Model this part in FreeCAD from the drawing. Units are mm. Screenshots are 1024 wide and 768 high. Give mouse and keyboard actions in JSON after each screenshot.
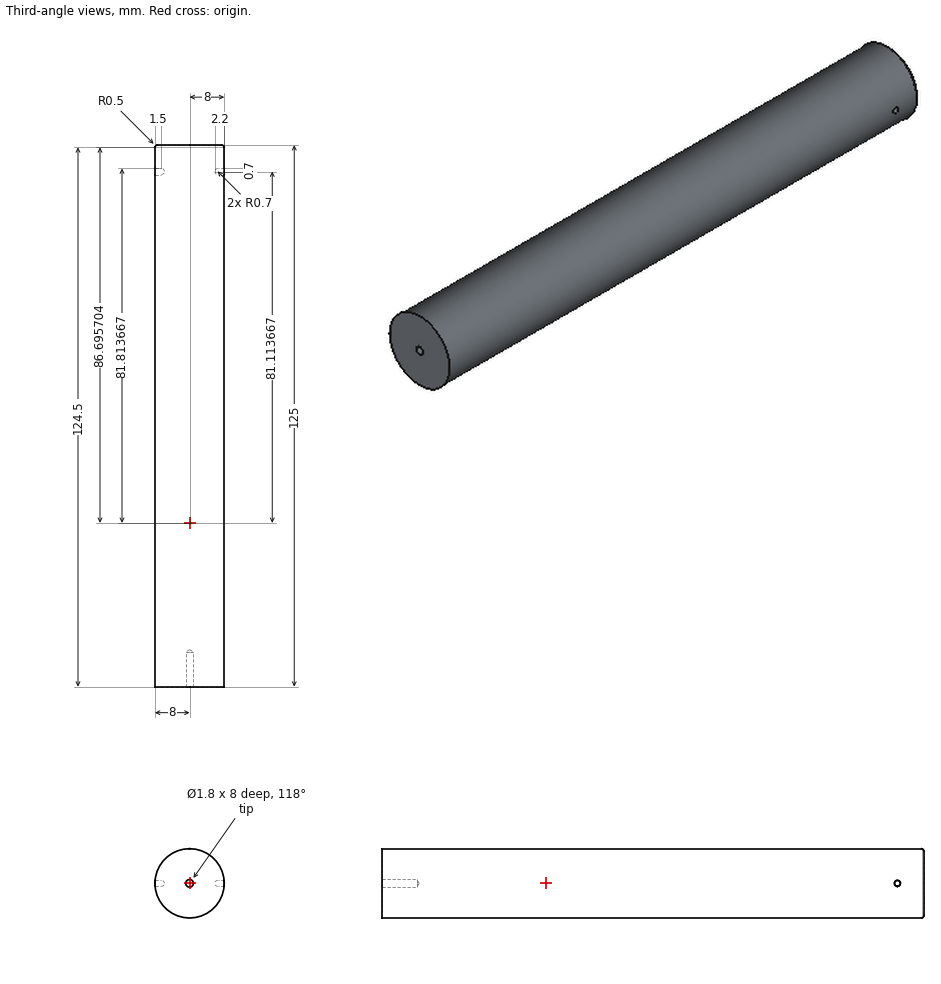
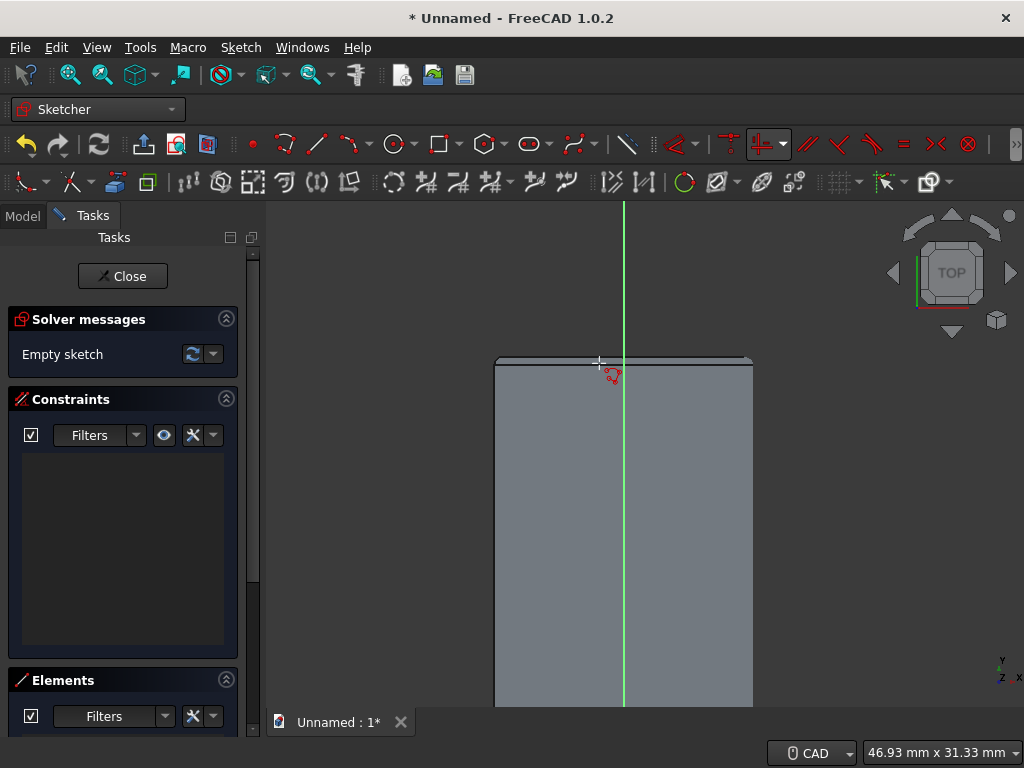
{"action": "left_click", "coordinate": [717, 455]}
{"action": "left_click", "coordinate": [753, 455]}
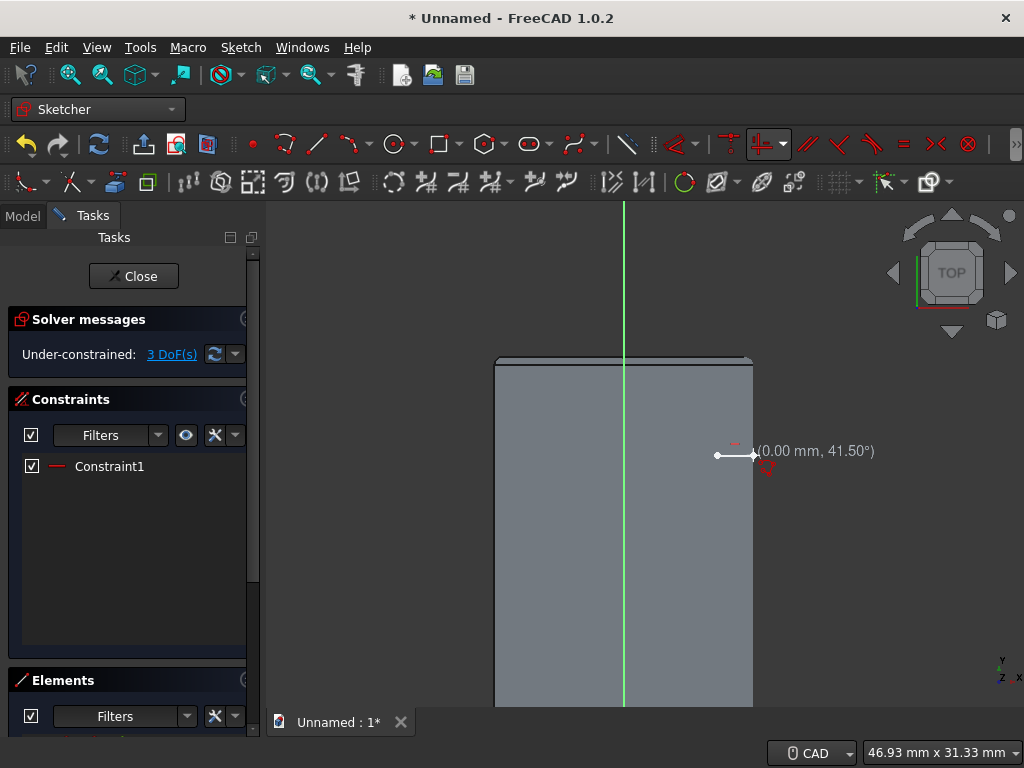
{"action": "scroll", "coordinate": [753, 444], "scroll_direction": "up", "scroll_amount": 2}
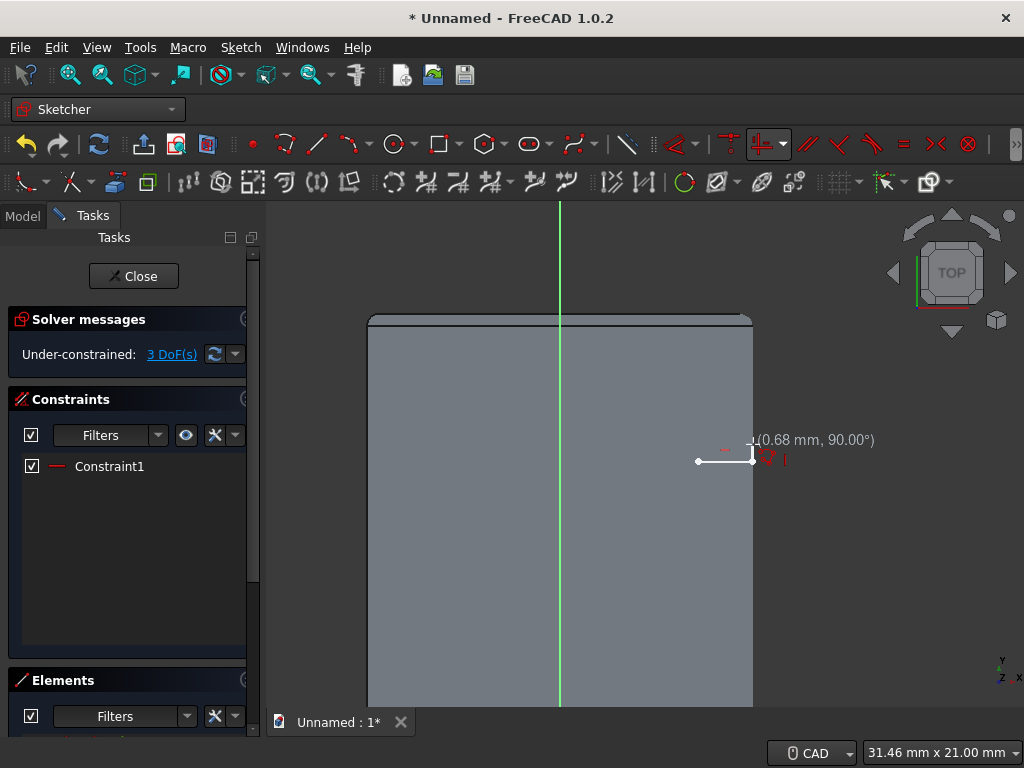
{"action": "left_click", "coordinate": [753, 443]}
{"action": "left_click", "coordinate": [716, 443]}
{"action": "right_click", "coordinate": [716, 443]}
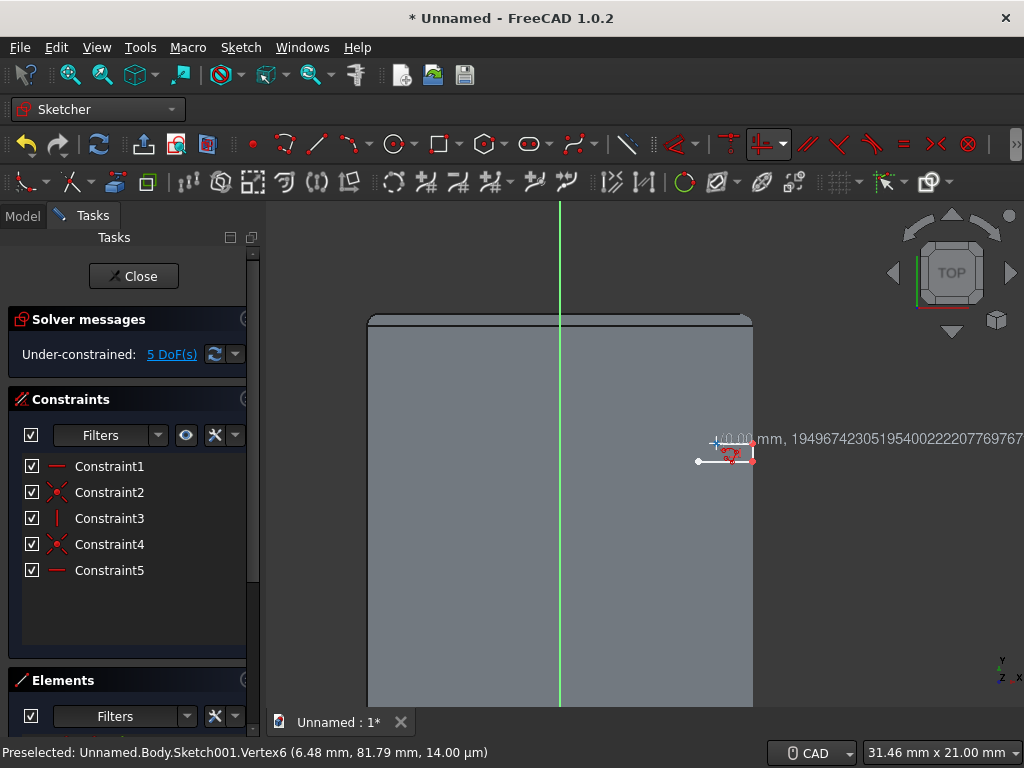
{"action": "key", "text": "g 3 a"}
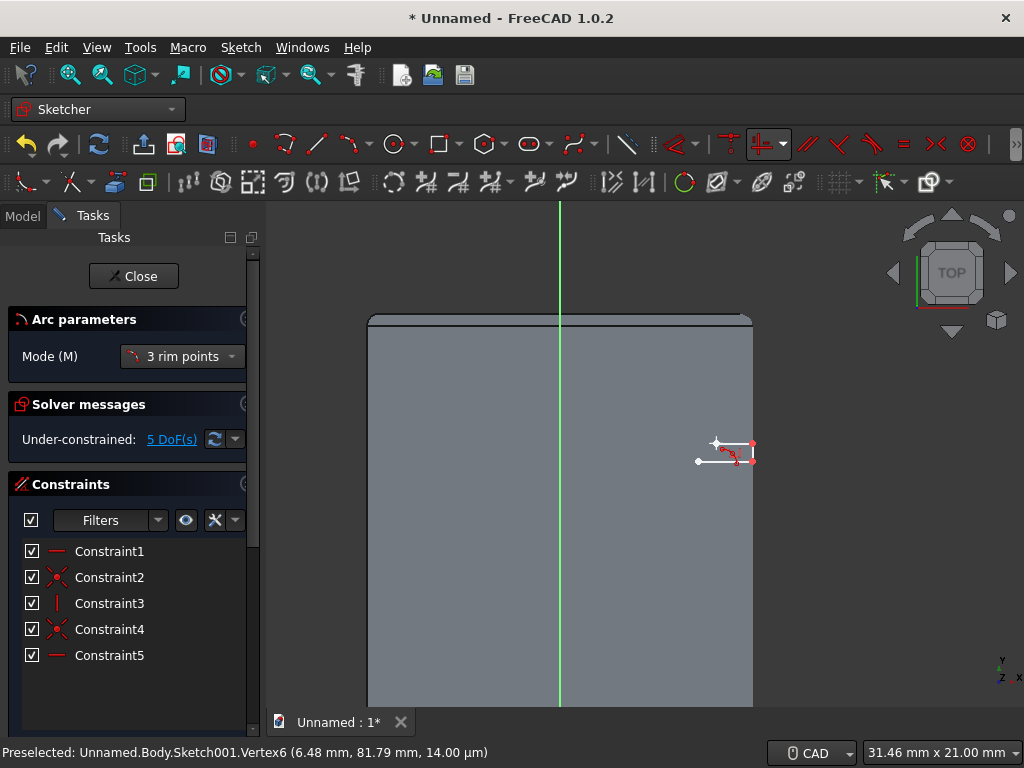
{"action": "left_click", "coordinate": [716, 444]}
{"action": "left_click", "coordinate": [699, 462]}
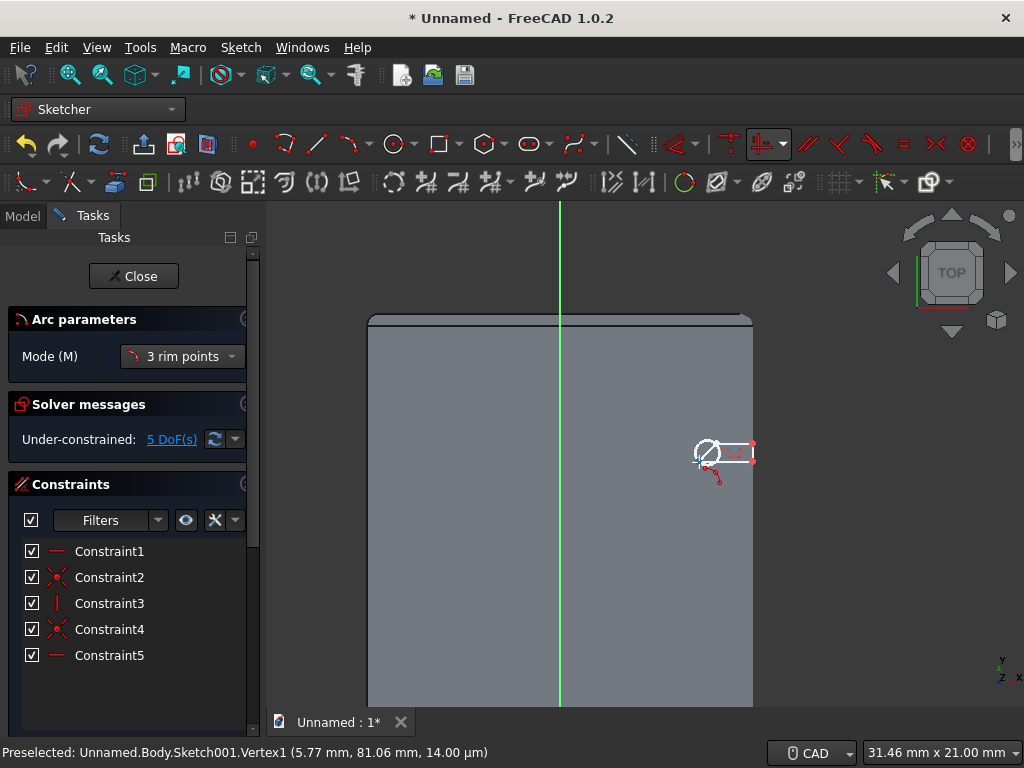
{"action": "scroll", "coordinate": [705, 448], "scroll_direction": "up", "scroll_amount": 6}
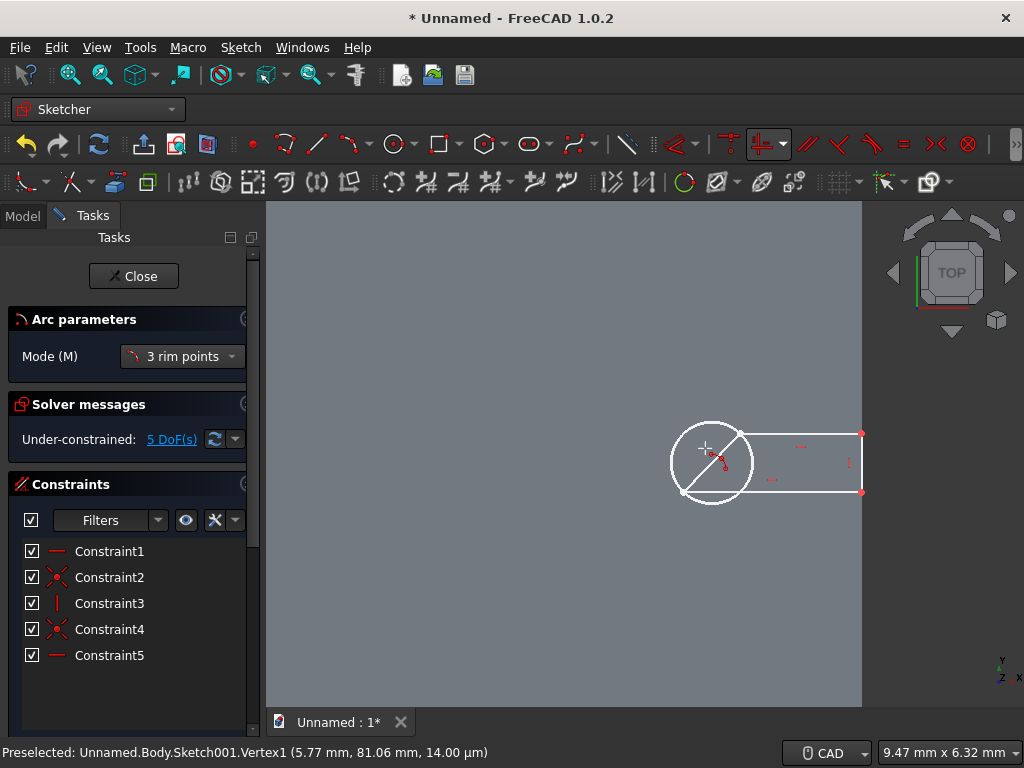
{"action": "left_click", "coordinate": [702, 448]}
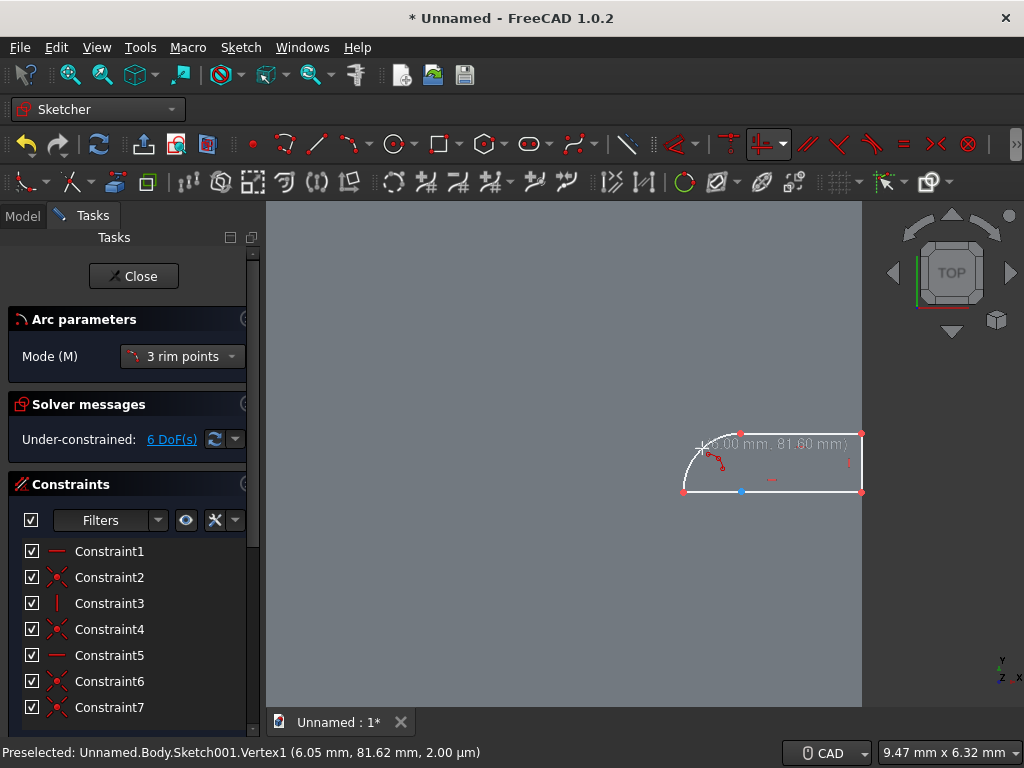
{"action": "key", "text": "g m"}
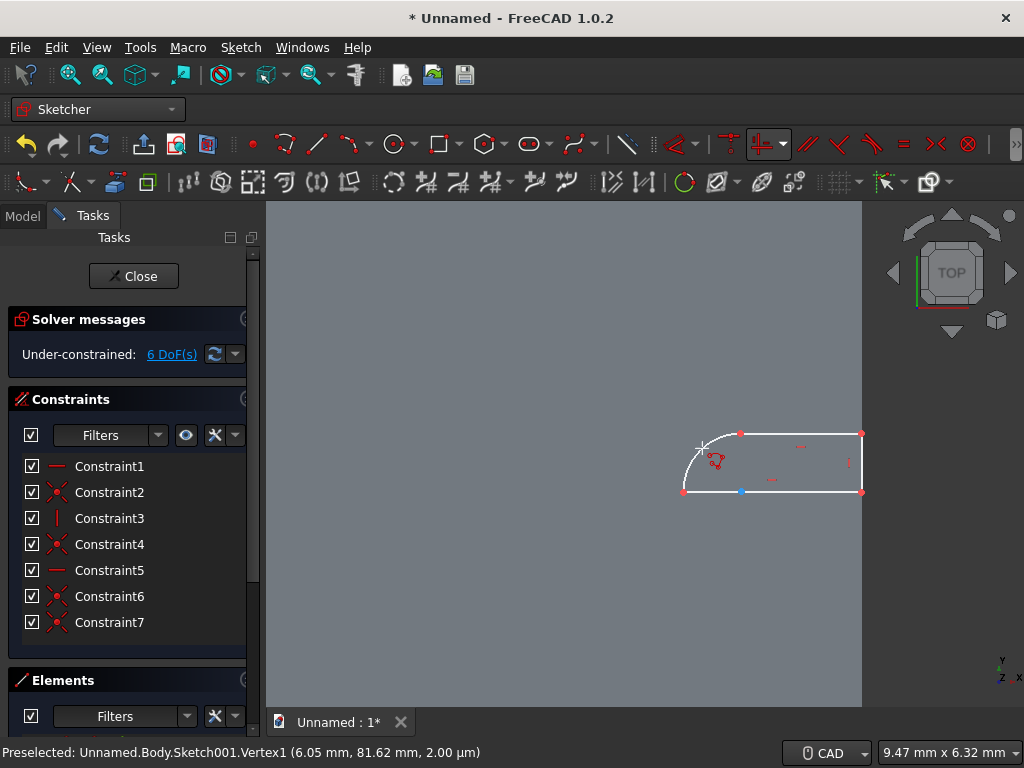
{"action": "scroll", "coordinate": [731, 453], "scroll_direction": "down", "scroll_amount": 8}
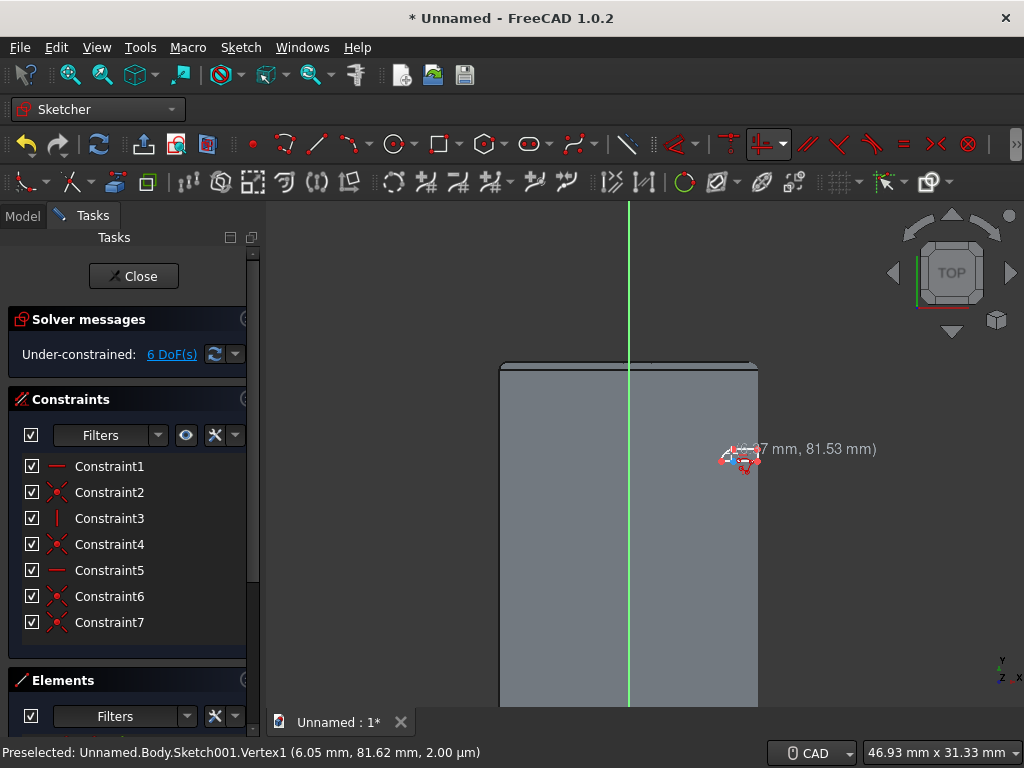
{"action": "left_click", "coordinate": [524, 449]}
{"action": "left_click", "coordinate": [499, 449]}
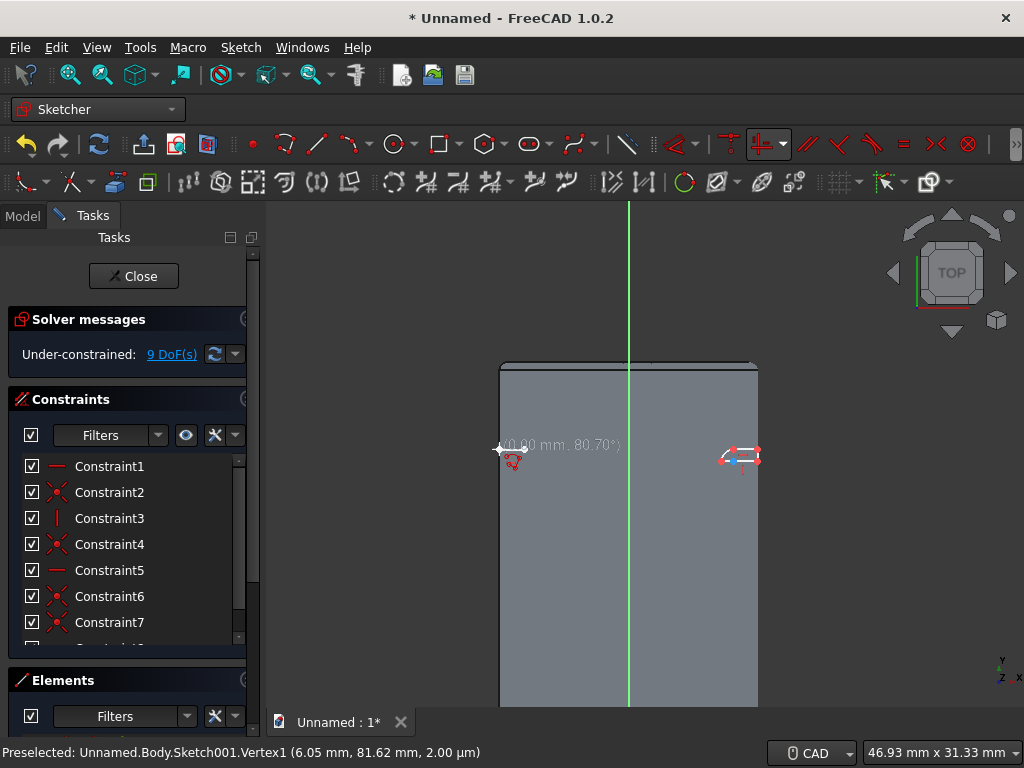
{"action": "scroll", "coordinate": [499, 460], "scroll_direction": "up", "scroll_amount": 2}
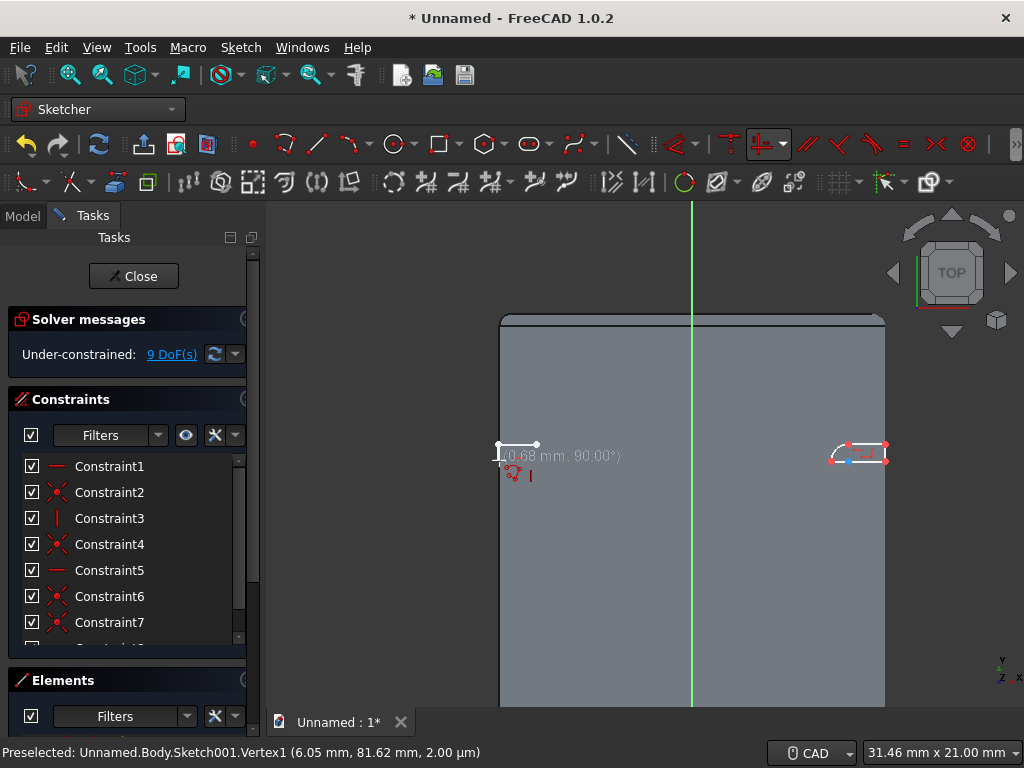
{"action": "left_click", "coordinate": [499, 460]}
{"action": "left_click", "coordinate": [553, 460]}
{"action": "right_click", "coordinate": [553, 460]}